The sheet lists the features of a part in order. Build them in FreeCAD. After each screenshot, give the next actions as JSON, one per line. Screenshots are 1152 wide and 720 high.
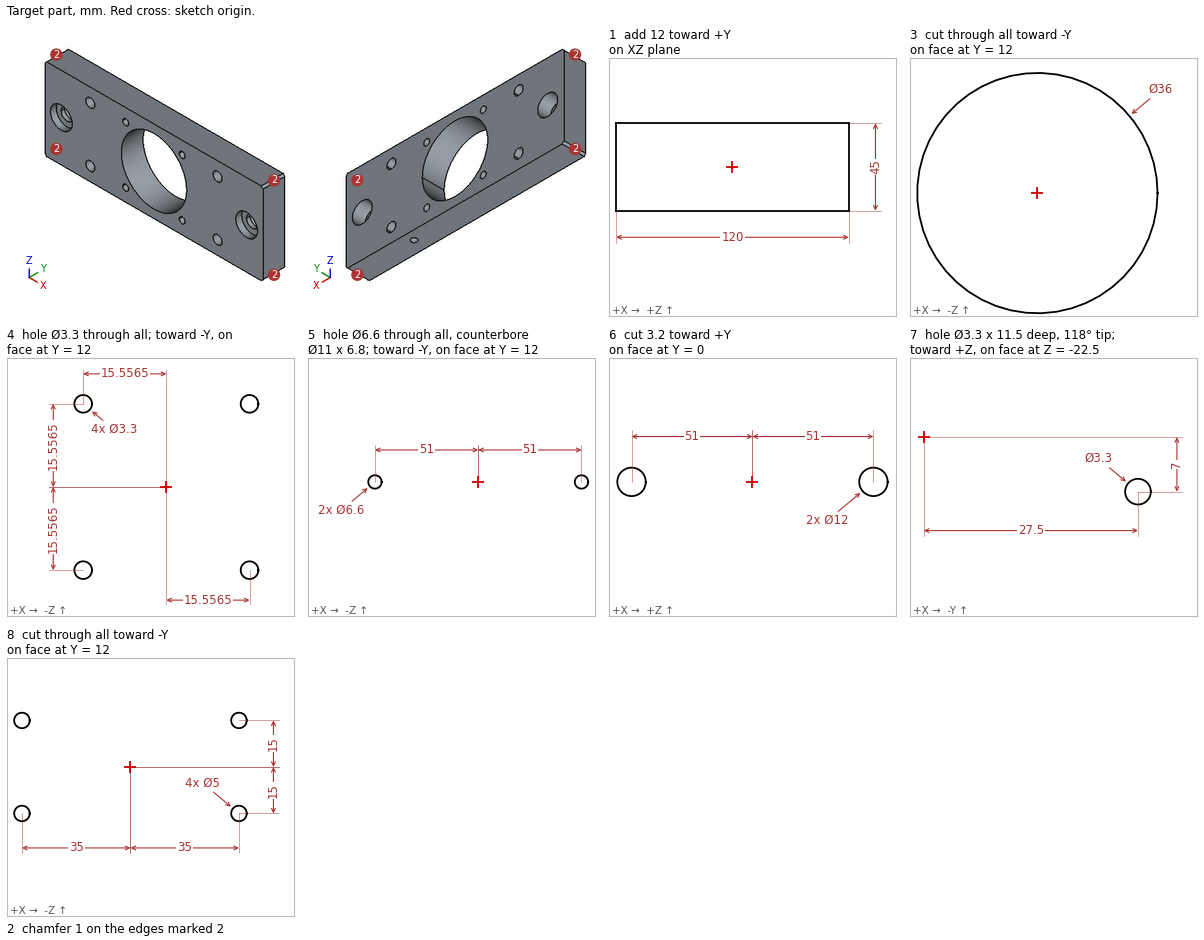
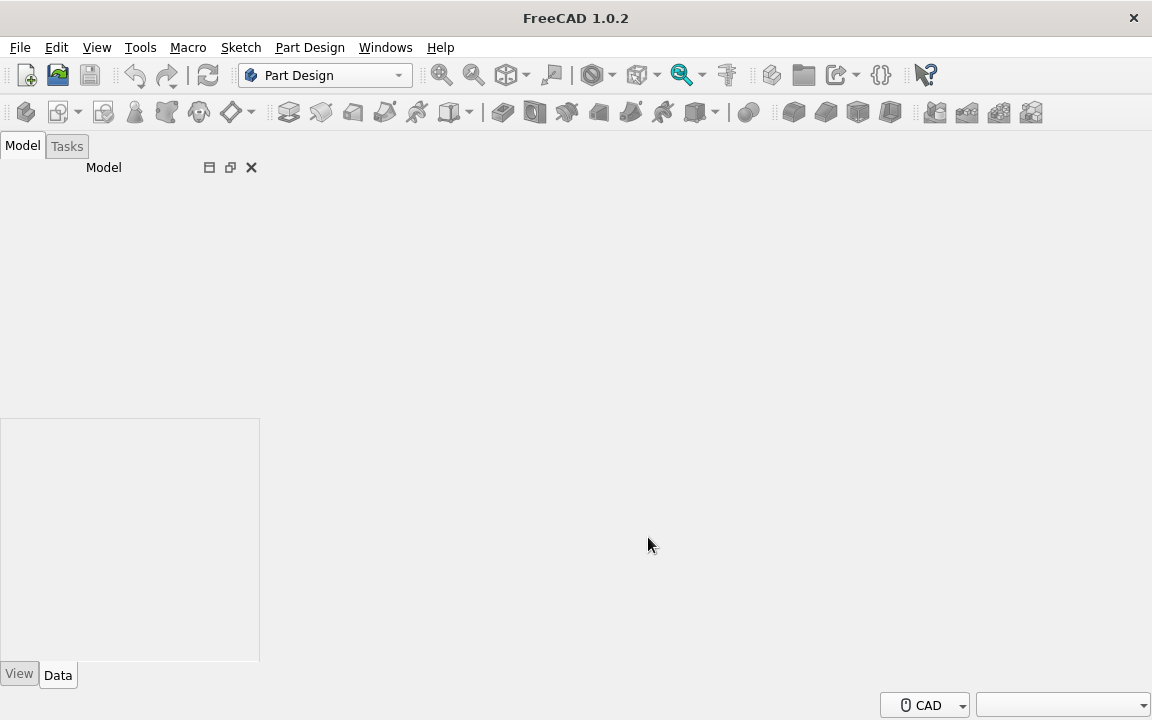
{"action": "left_click", "coordinate": [26, 76]}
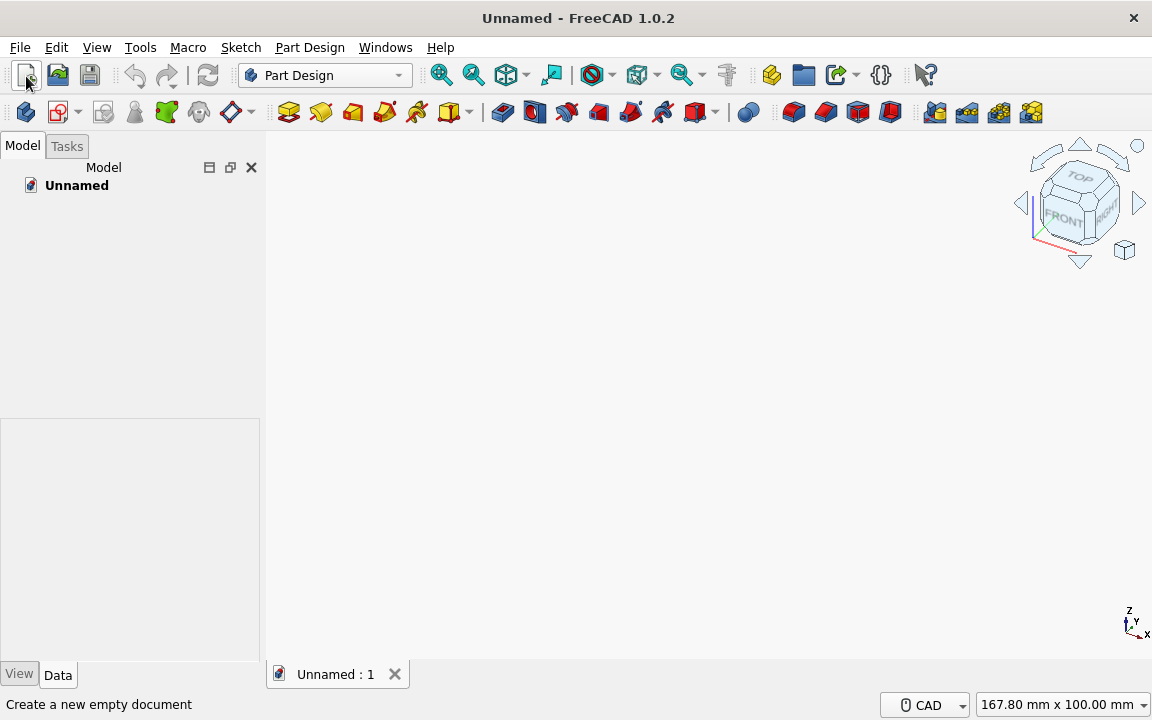
{"action": "left_click", "coordinate": [58, 112]}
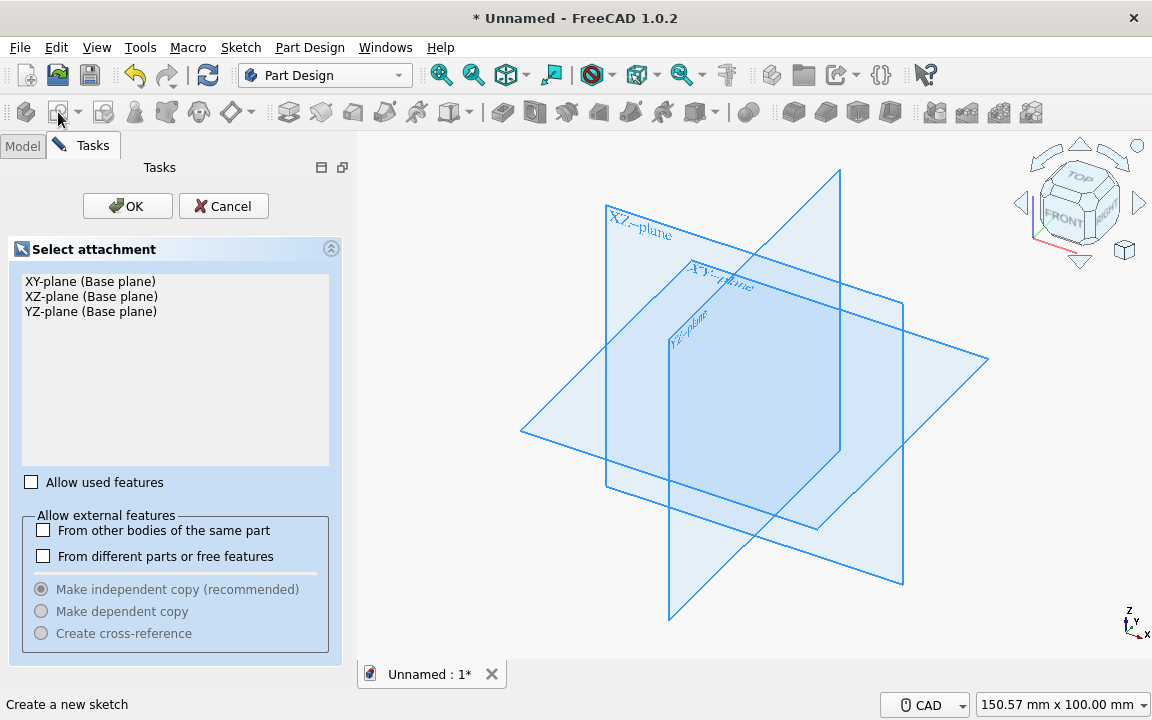
{"action": "left_click", "coordinate": [82, 296]}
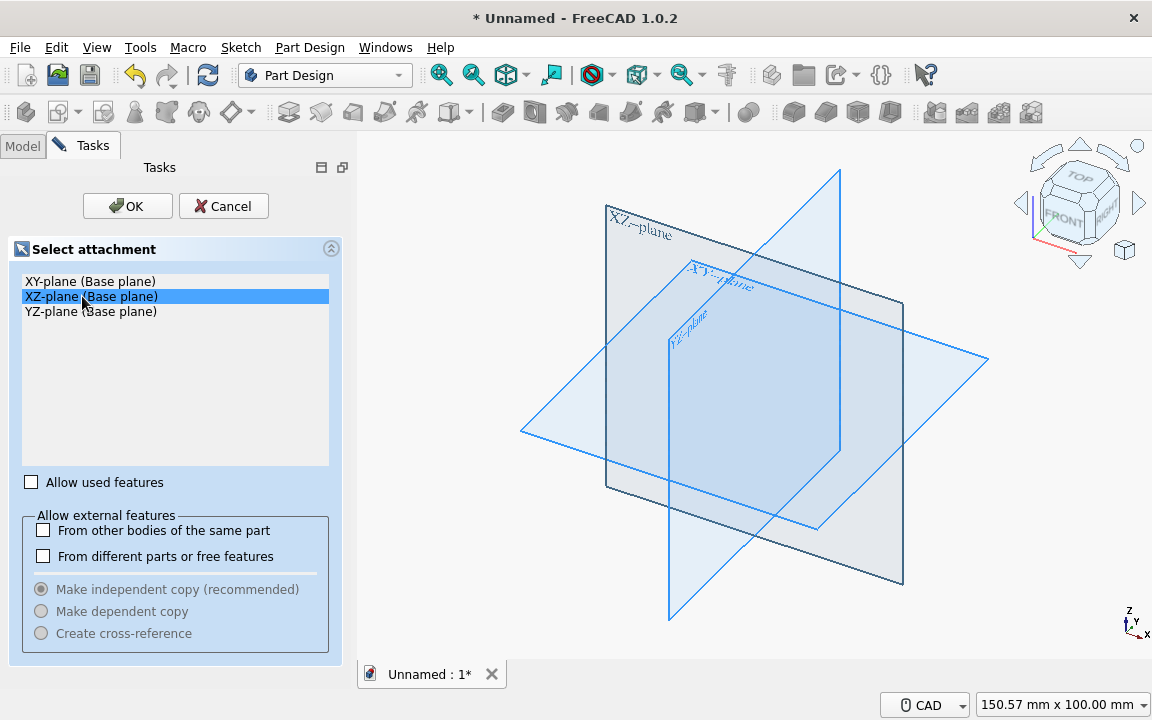
{"action": "left_click", "coordinate": [128, 206]}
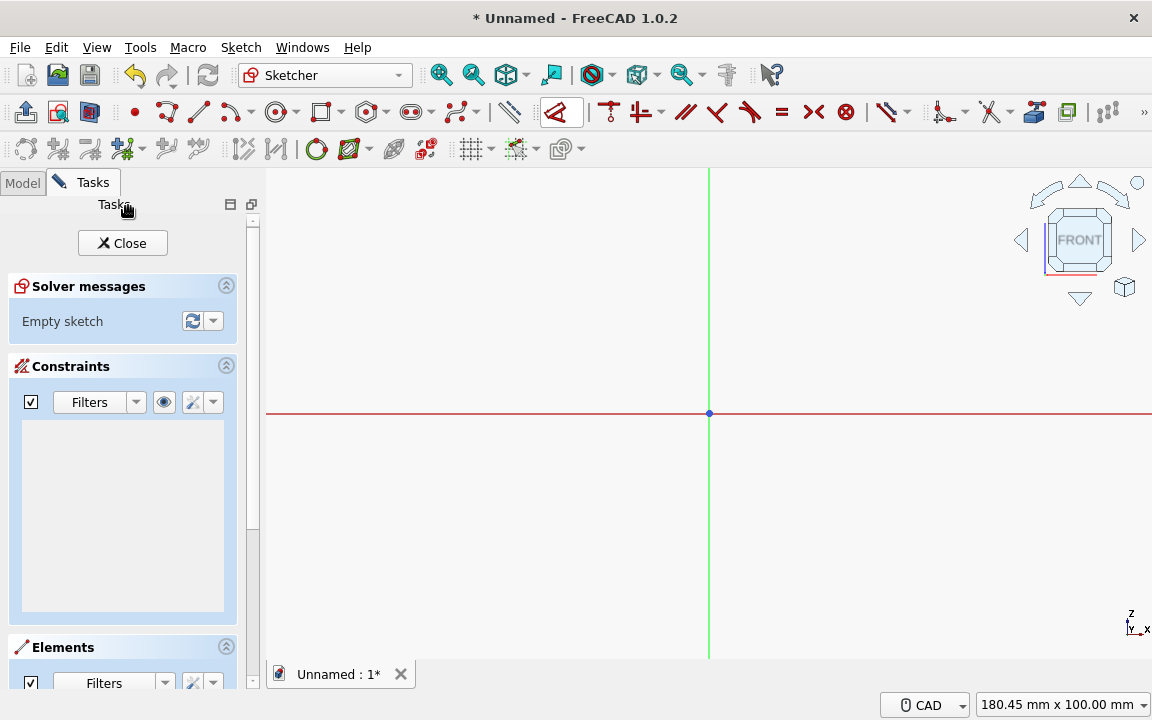
{"action": "scroll", "coordinate": [331, 413], "scroll_direction": "down", "scroll_amount": 1}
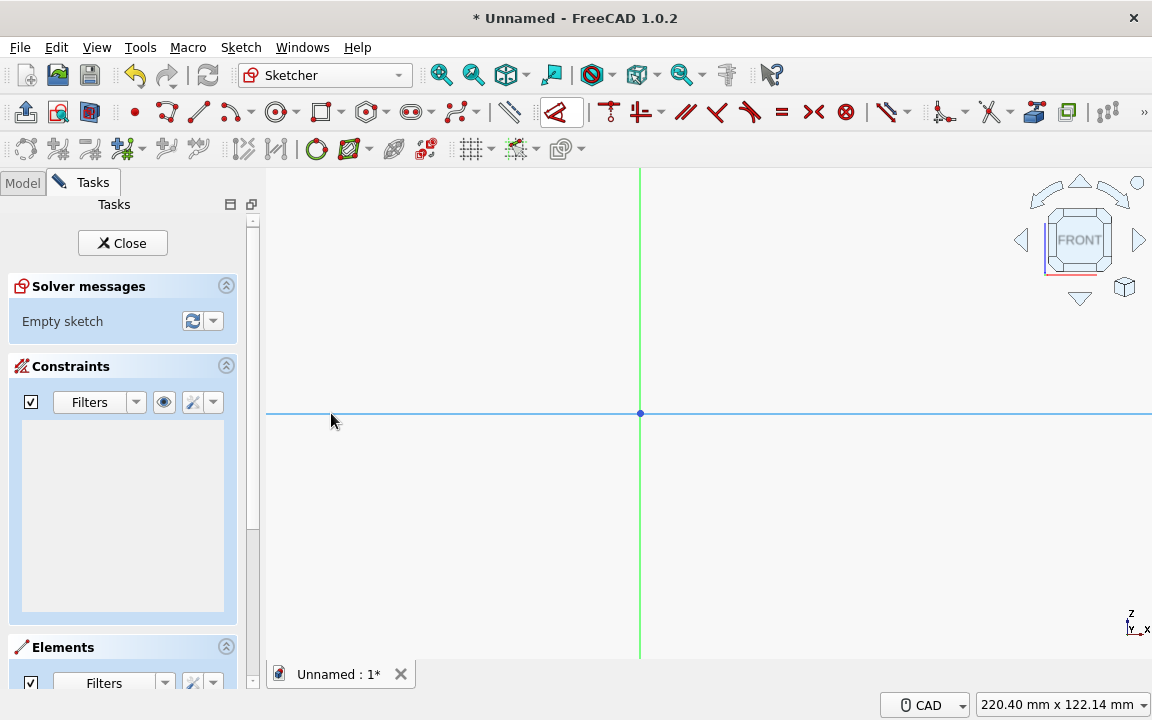
{"action": "left_click", "coordinate": [344, 112]}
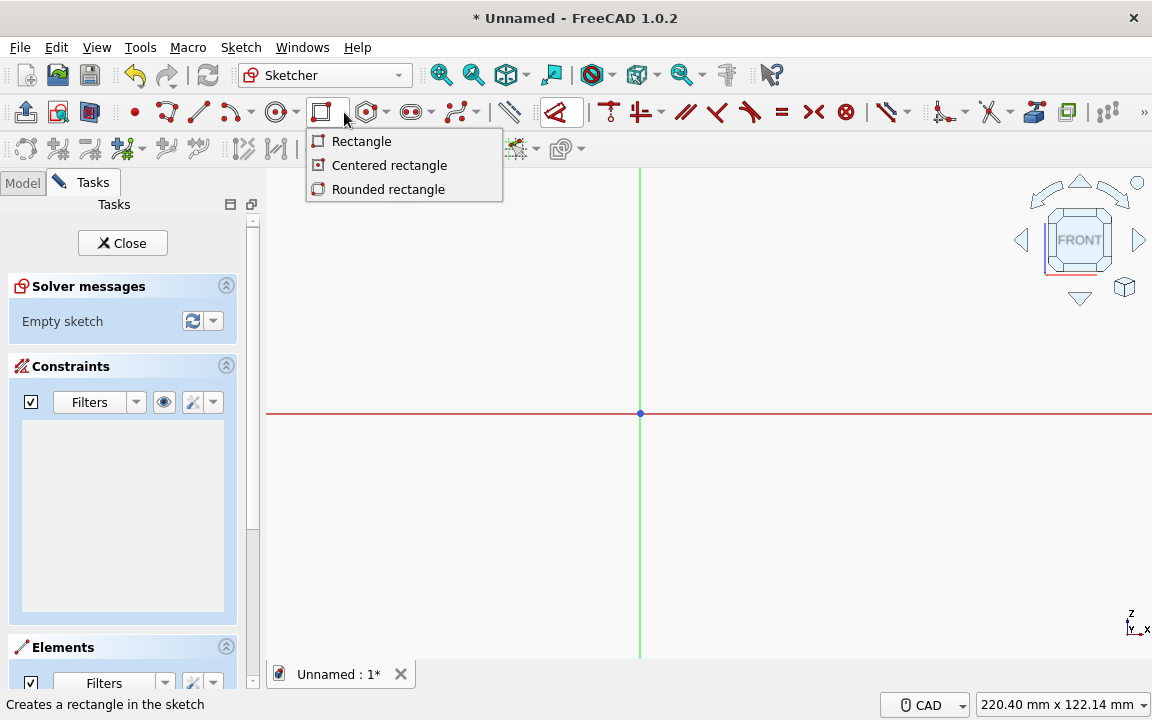
{"action": "left_click", "coordinate": [404, 165]}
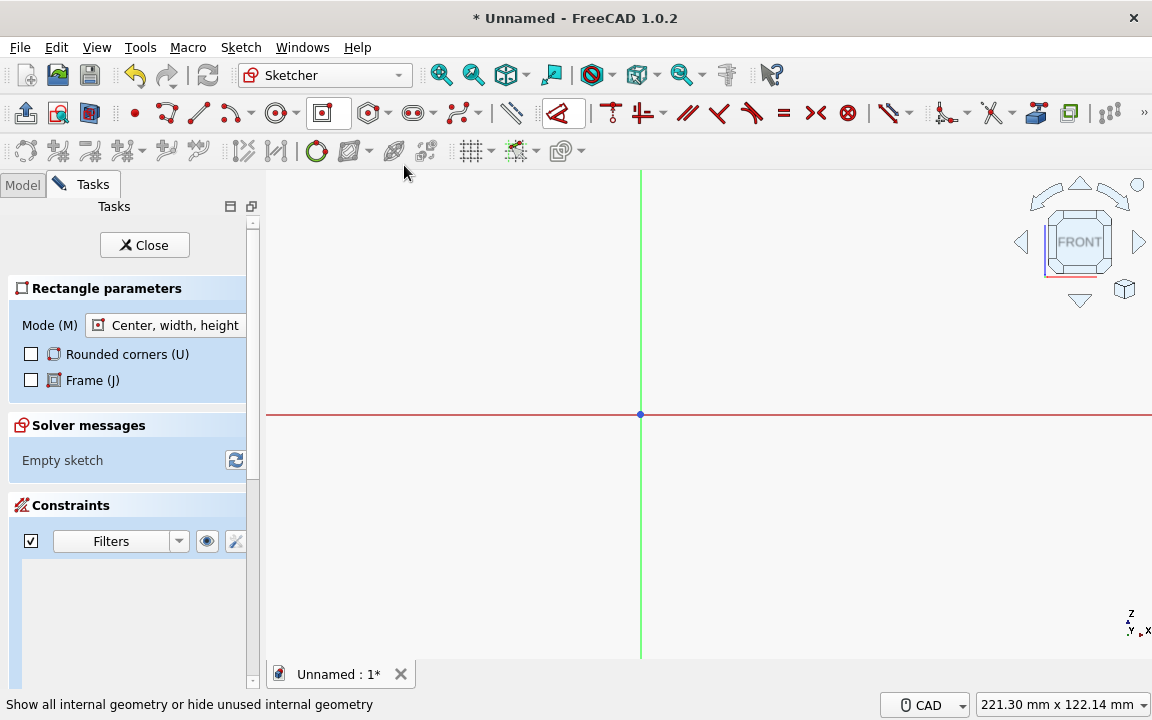
{"action": "left_click", "coordinate": [641, 414]}
{"action": "mouse_move", "coordinate": [881, 324]}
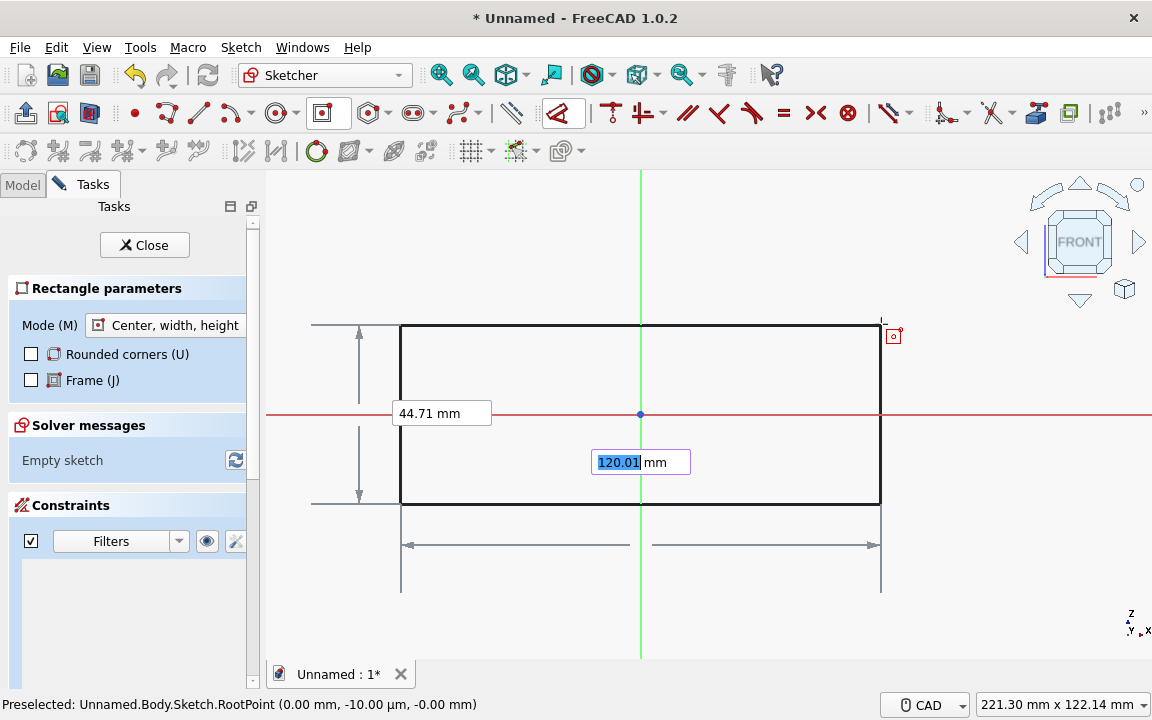
{"action": "type", "text": "120"}
{"action": "key", "text": "Tab"}
{"action": "type", "text": "45"}
{"action": "key", "text": "Return"}
{"action": "key", "text": "Escape"}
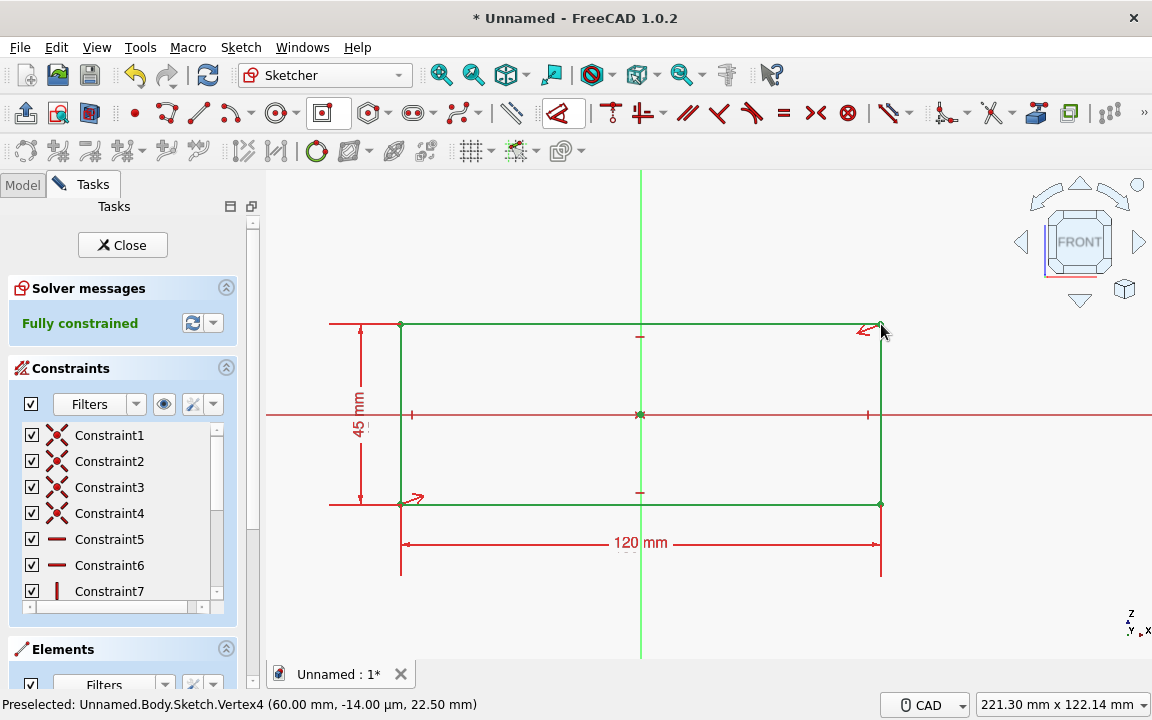
{"action": "left_click", "coordinate": [123, 245]}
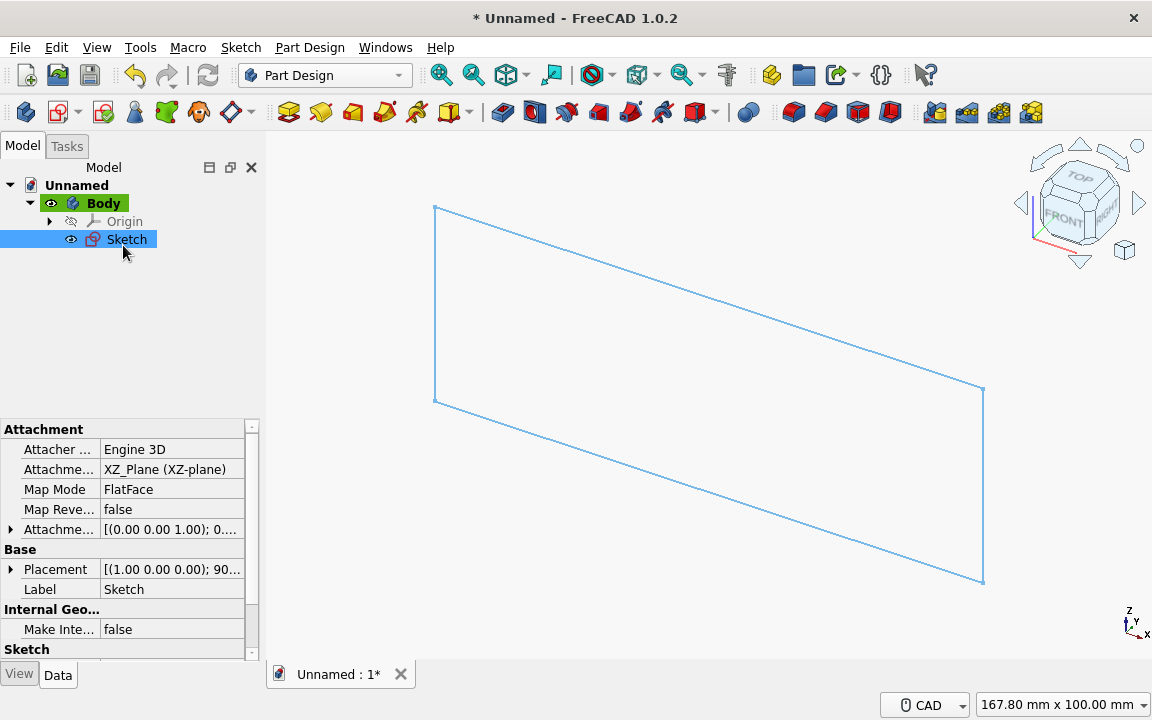
{"action": "left_click", "coordinate": [290, 112]}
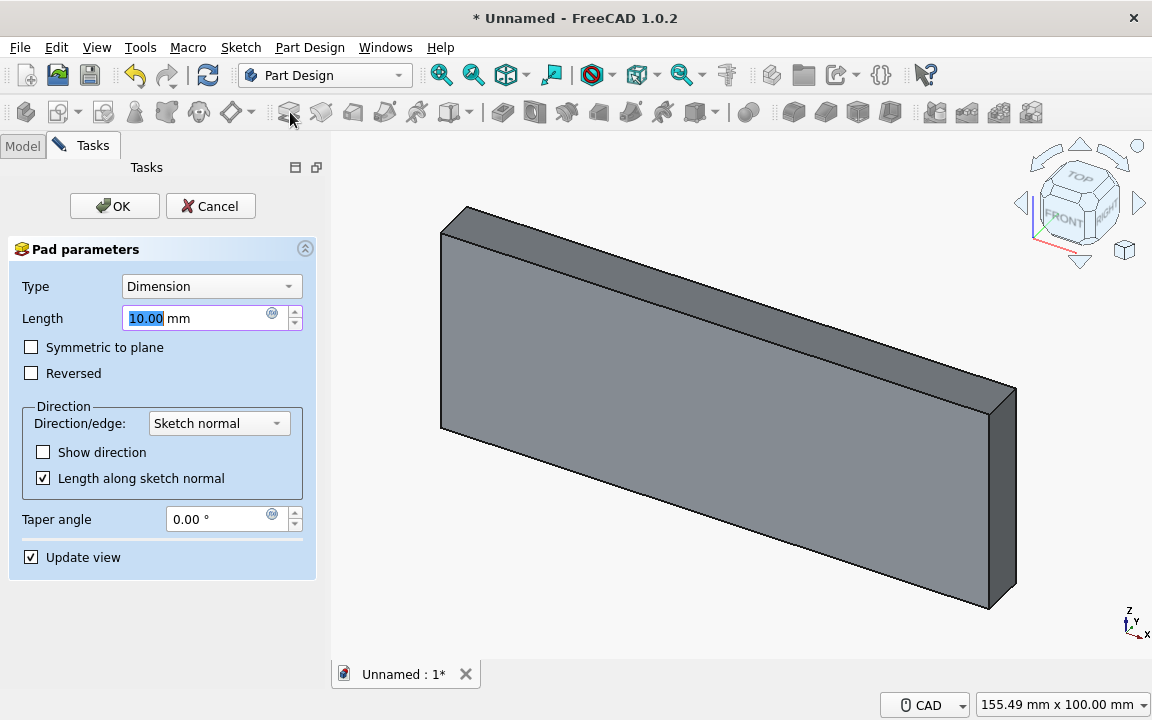
{"action": "type", "text": "12"}
{"action": "key", "text": "Tab"}